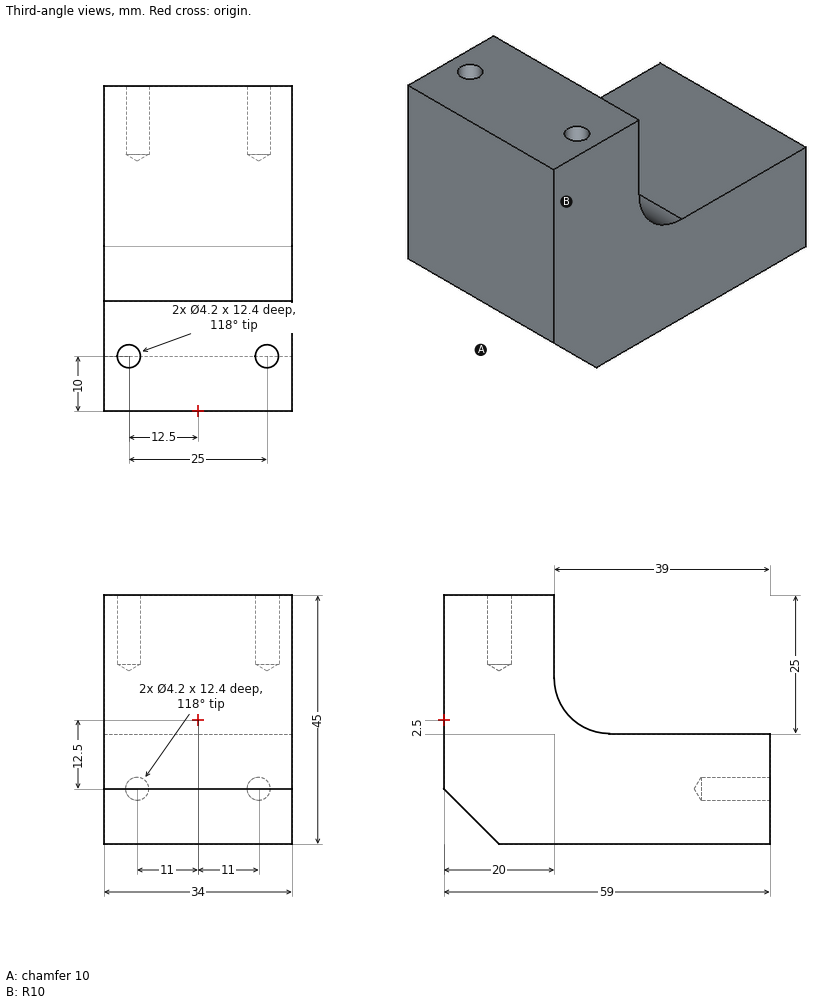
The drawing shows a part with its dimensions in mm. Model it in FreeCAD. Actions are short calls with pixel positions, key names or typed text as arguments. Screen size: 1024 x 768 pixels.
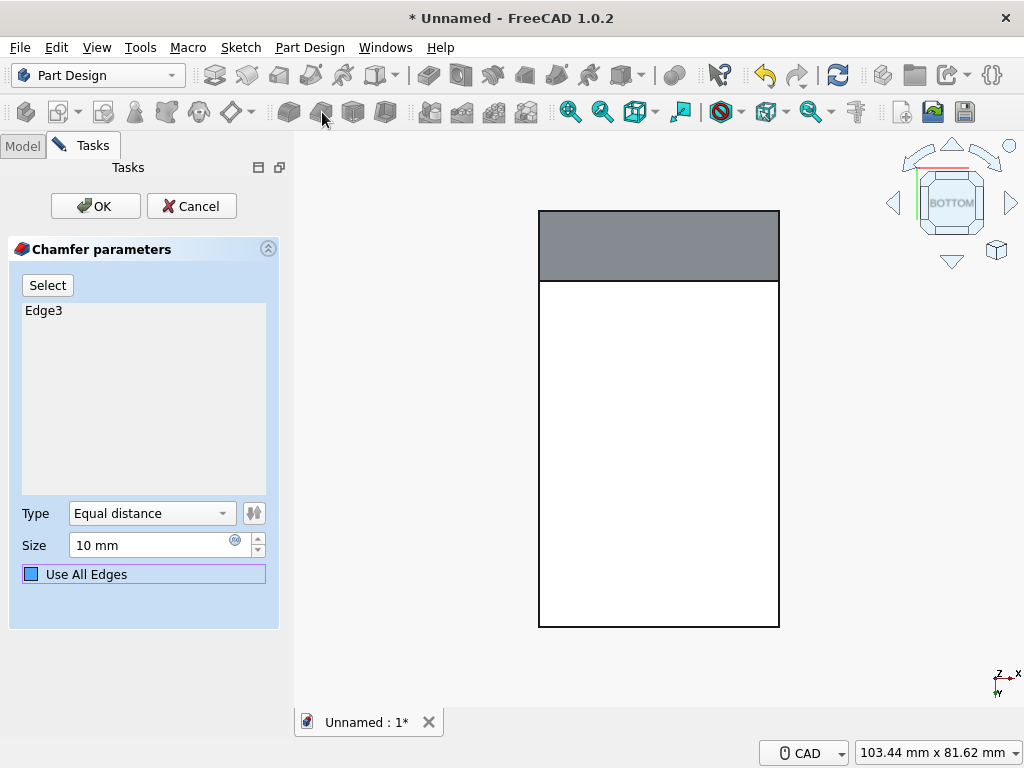
click(96, 206)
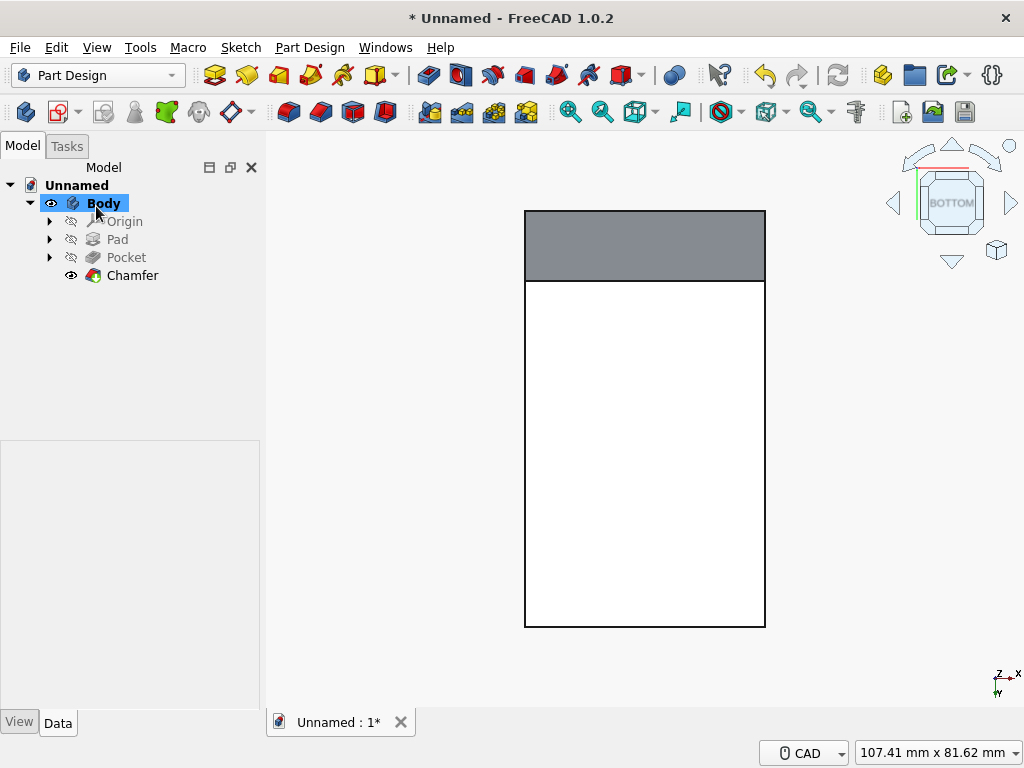
key(0)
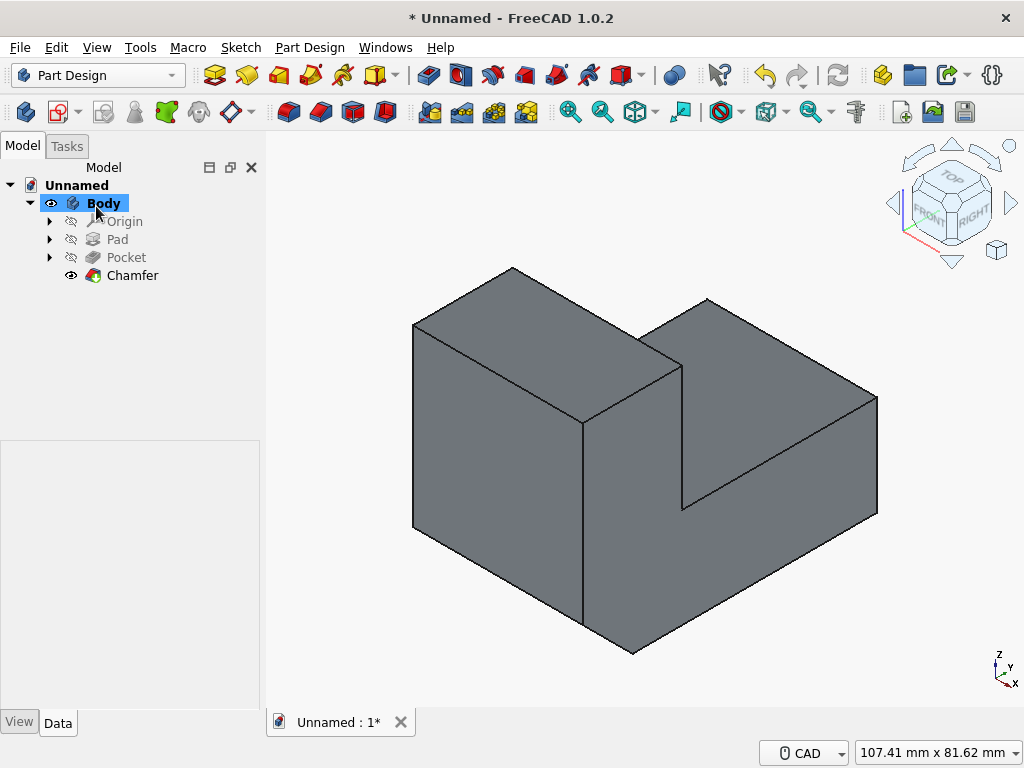
key(2)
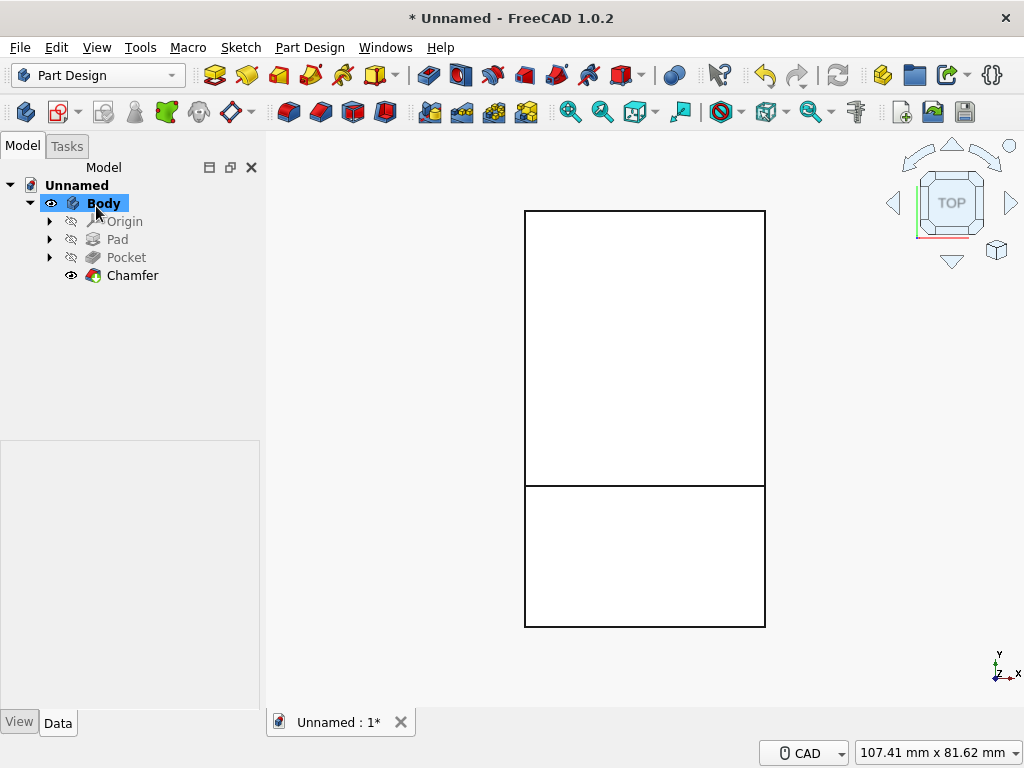
key(1)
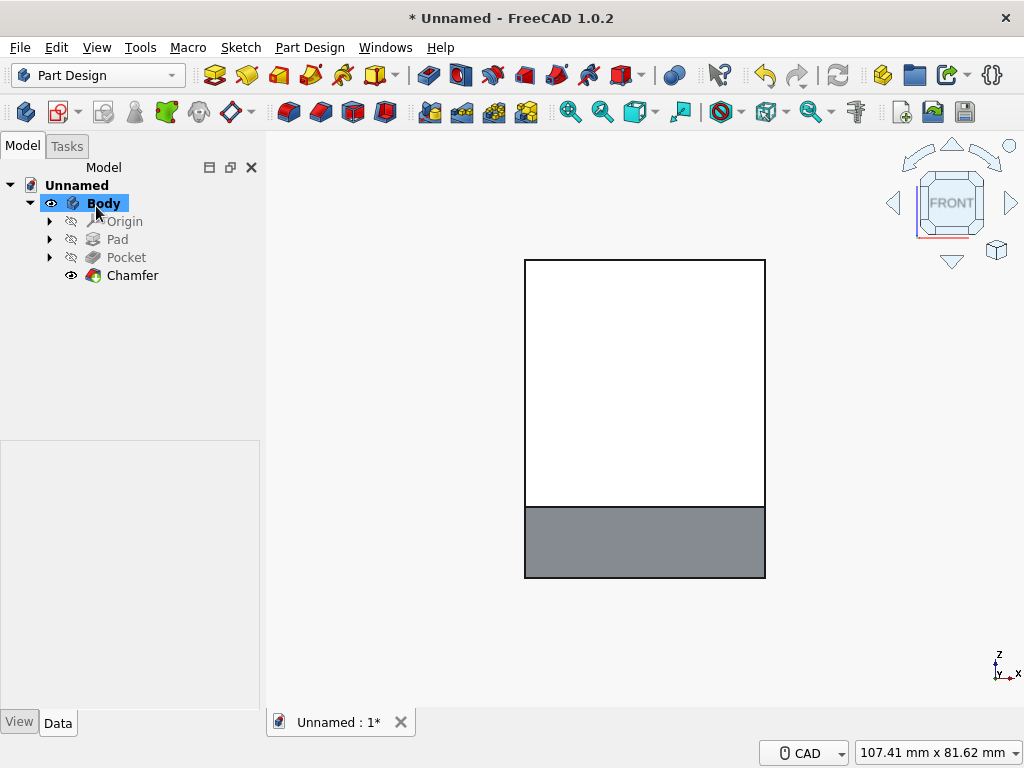
key(3)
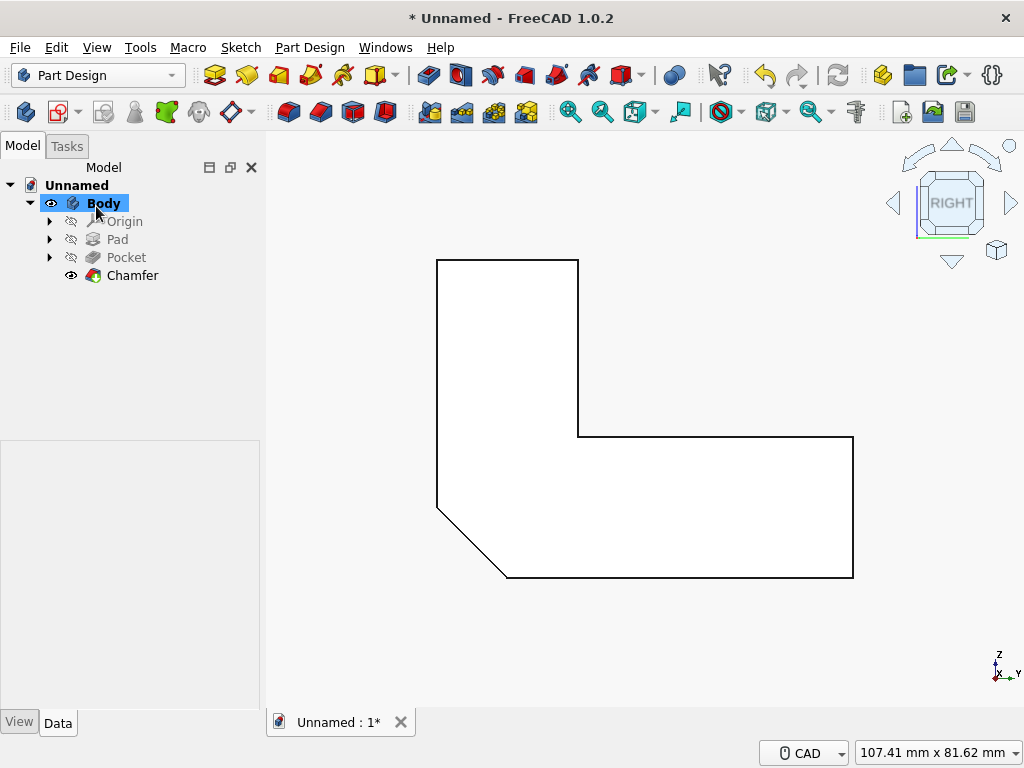
key(5)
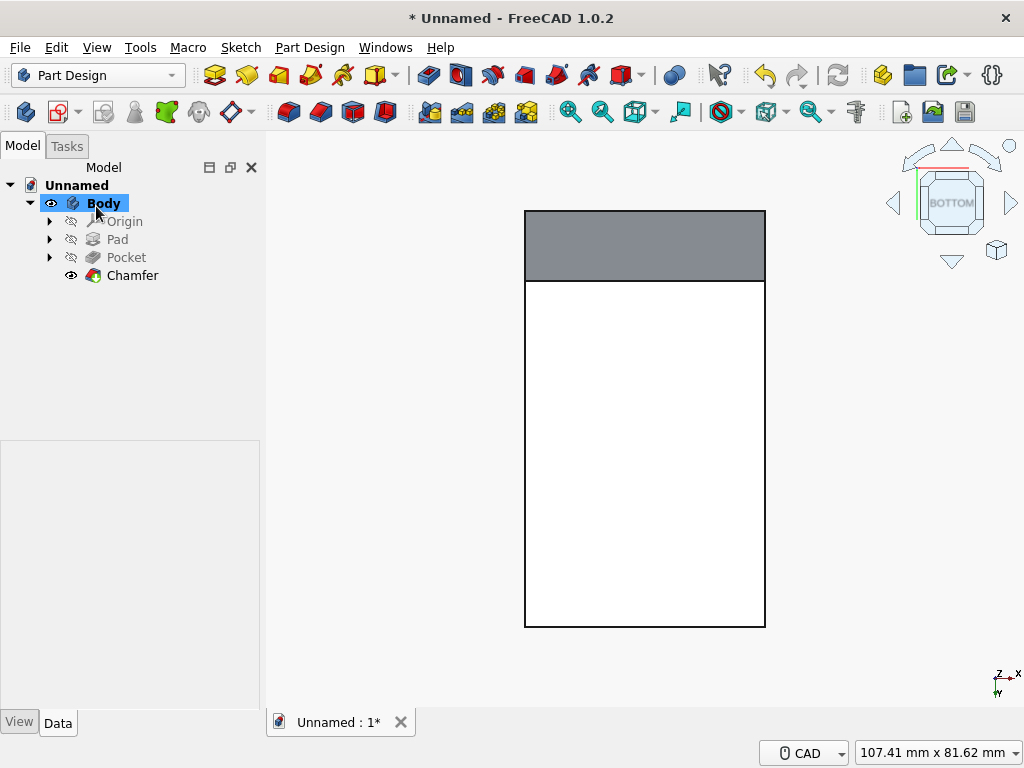
key(4)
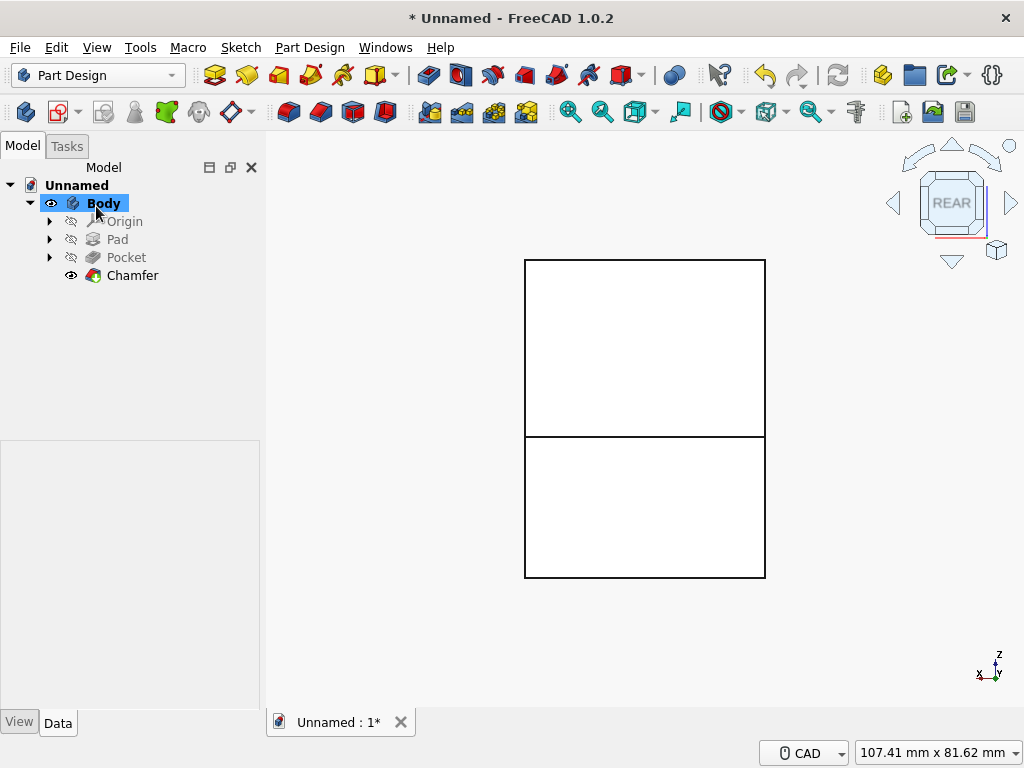
key(6)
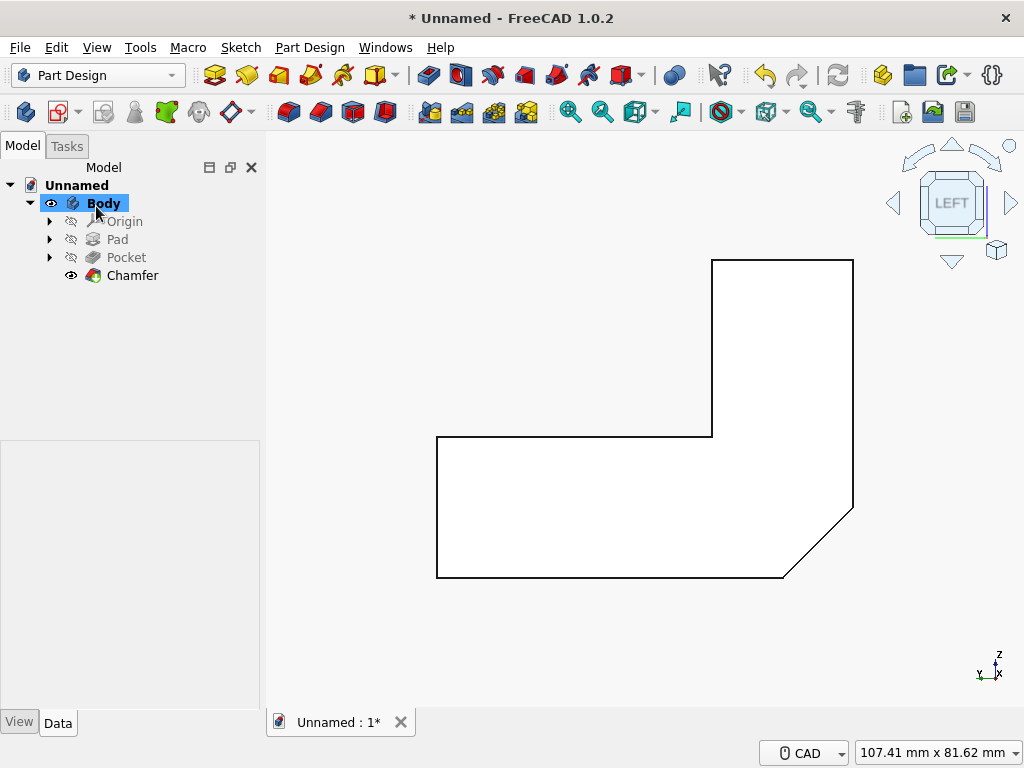
key(v)
key(3)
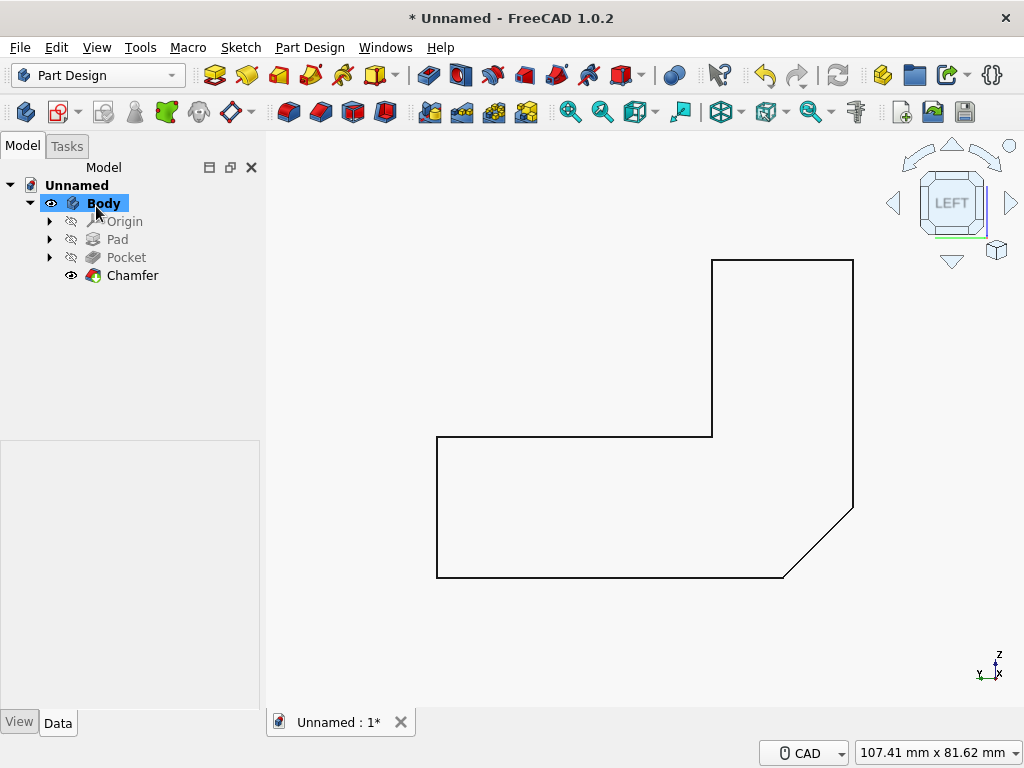
key(0)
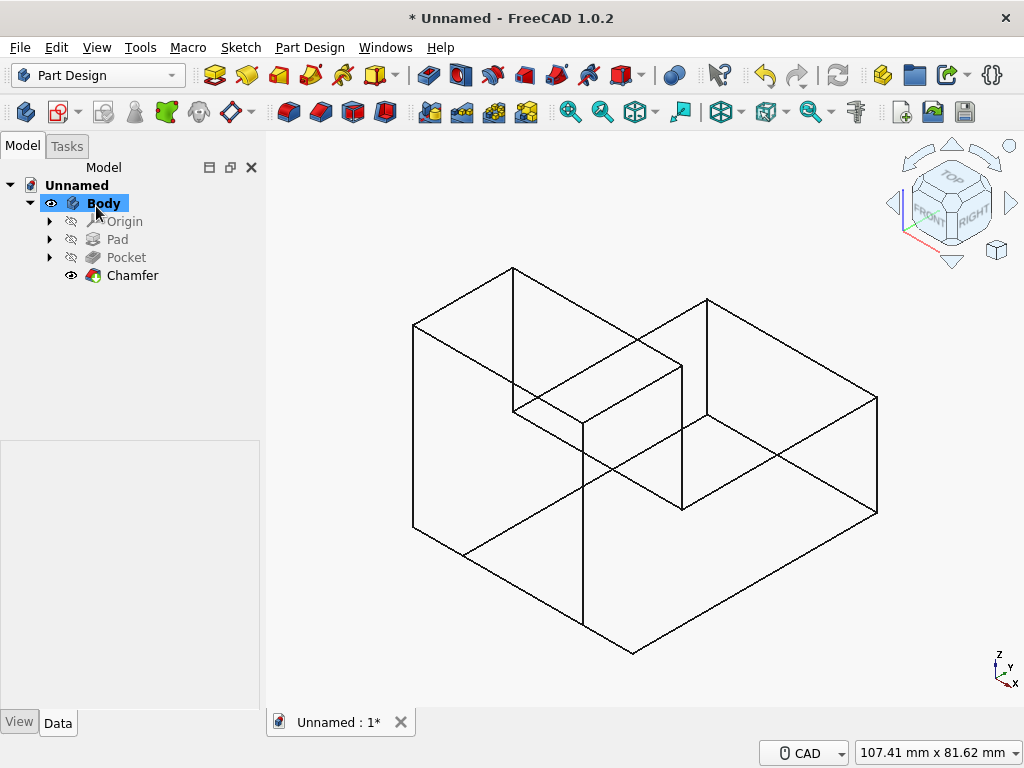
click(598, 460)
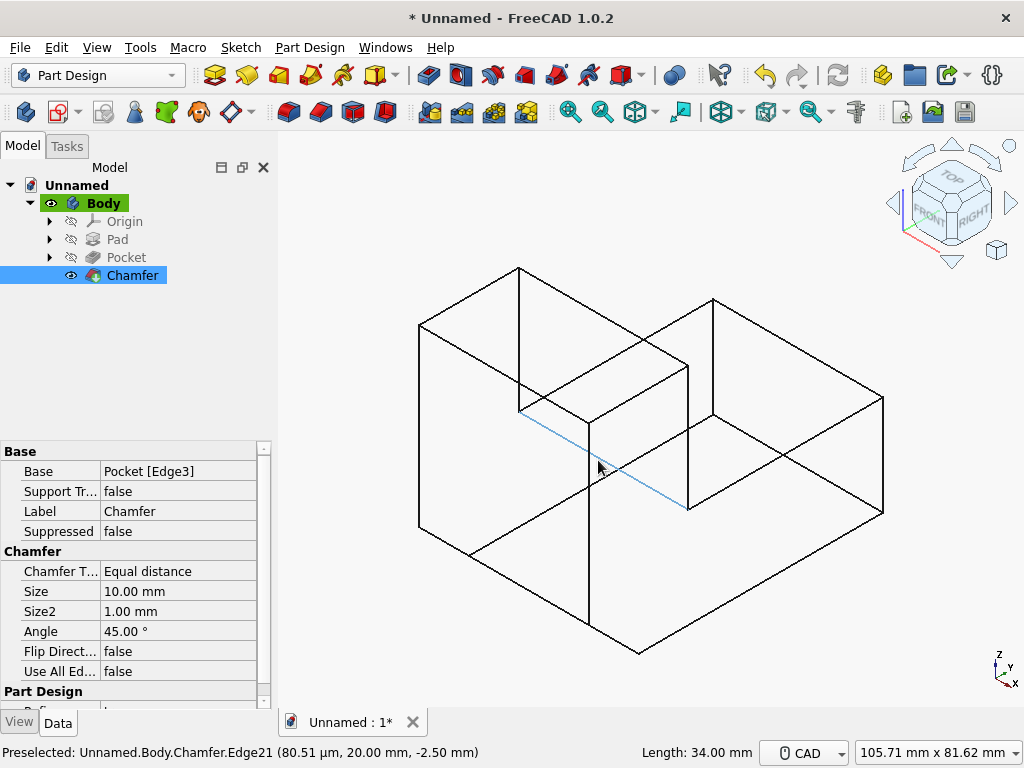
key(v)
key(1)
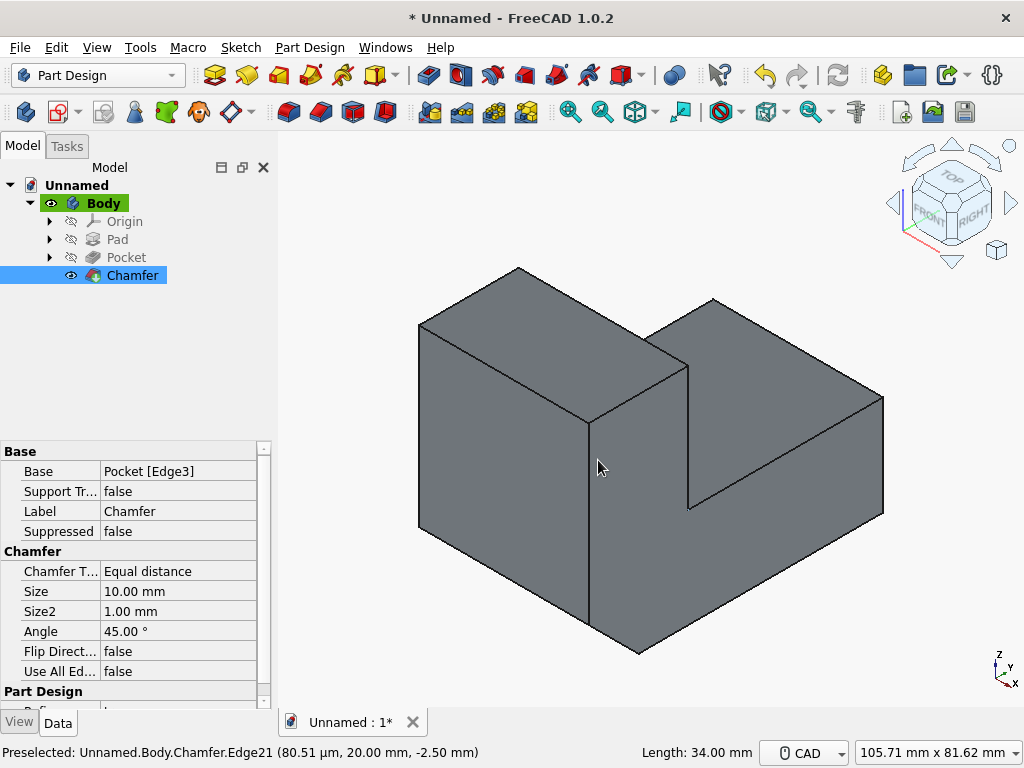
click(290, 112)